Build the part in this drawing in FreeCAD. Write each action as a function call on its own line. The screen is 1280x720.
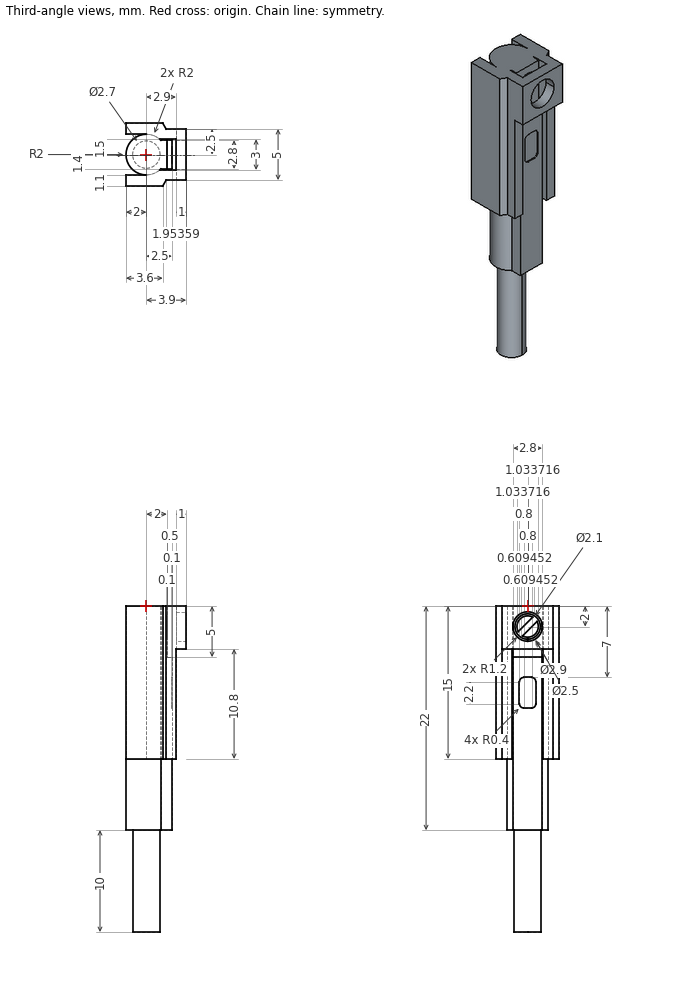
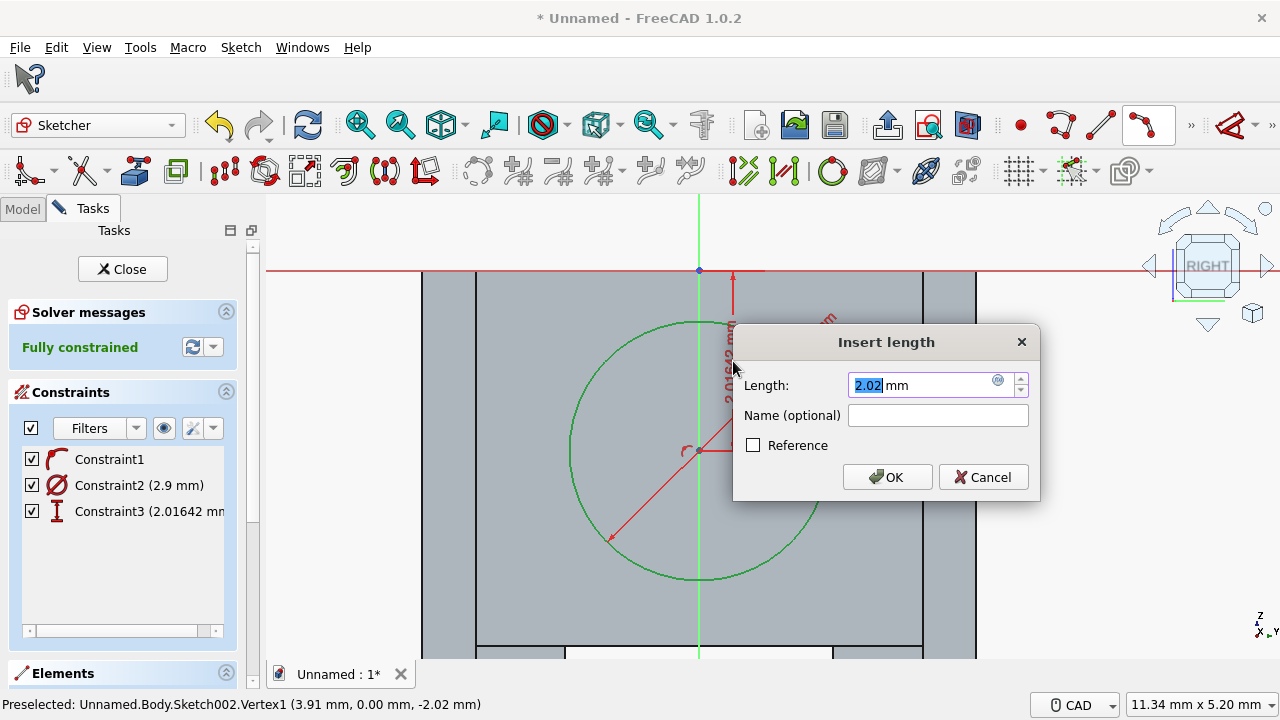
text(2)
key(Return)
key(Escape)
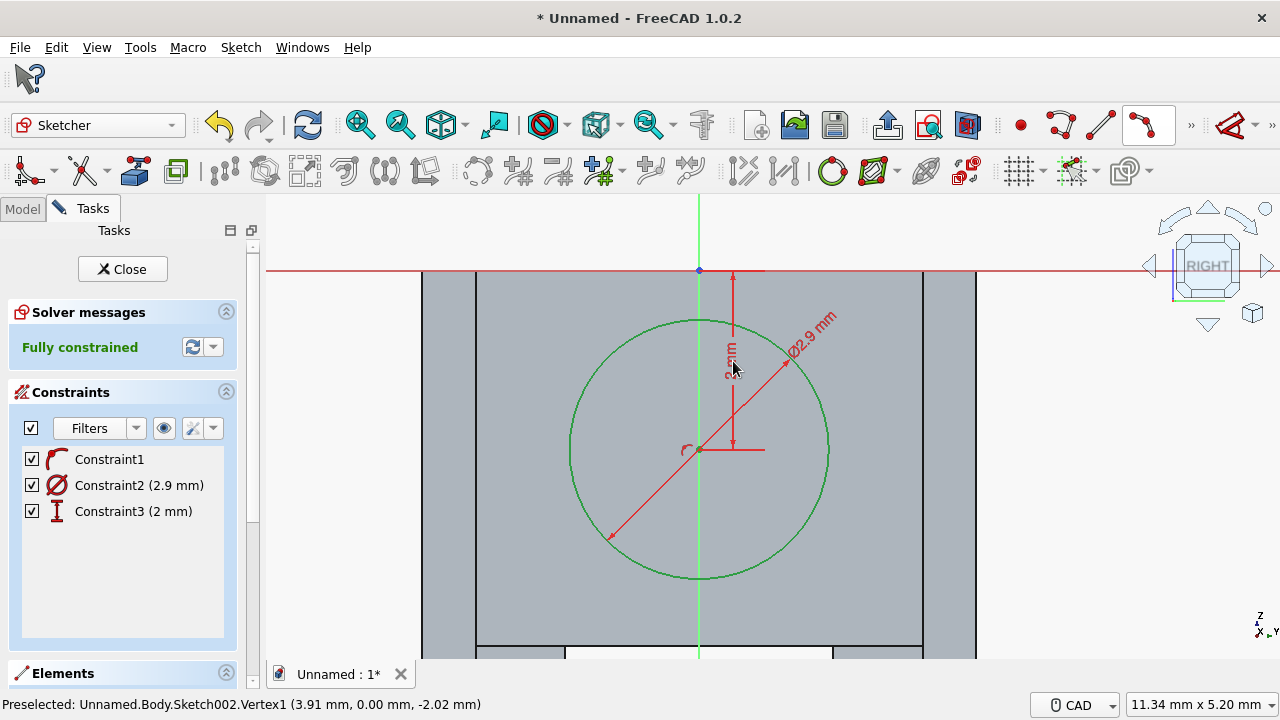
click(123, 269)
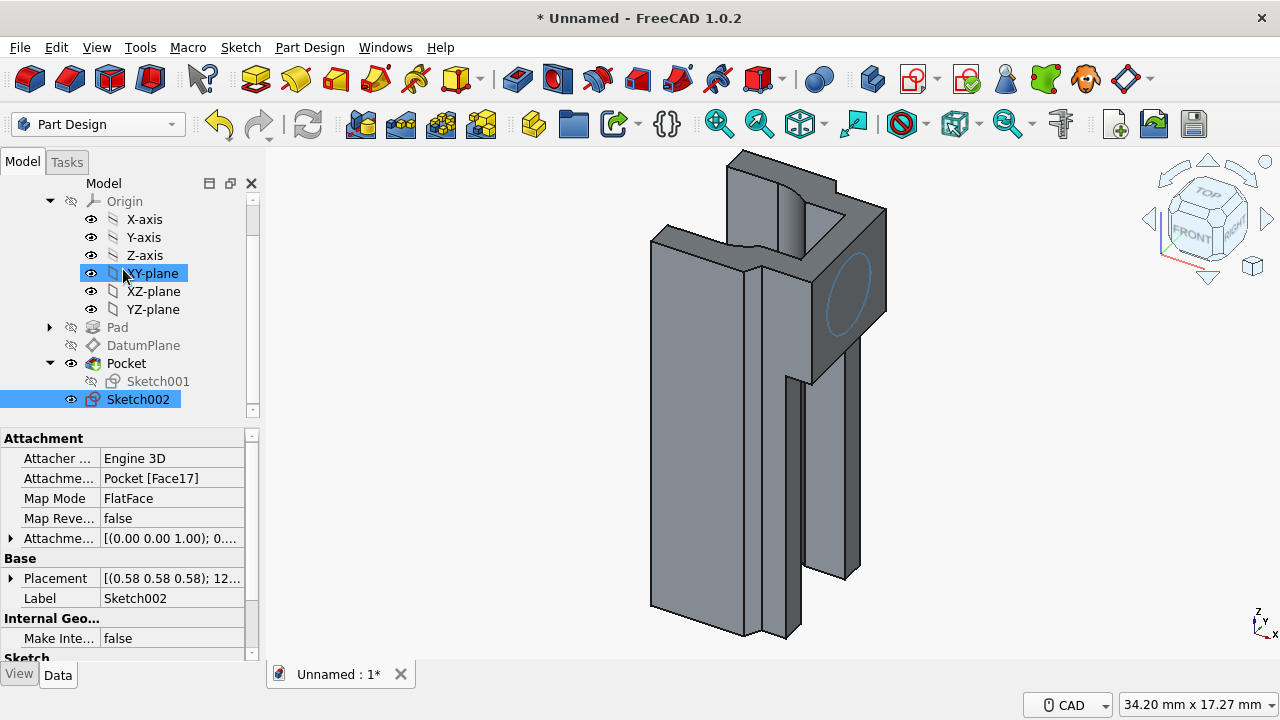
click(518, 80)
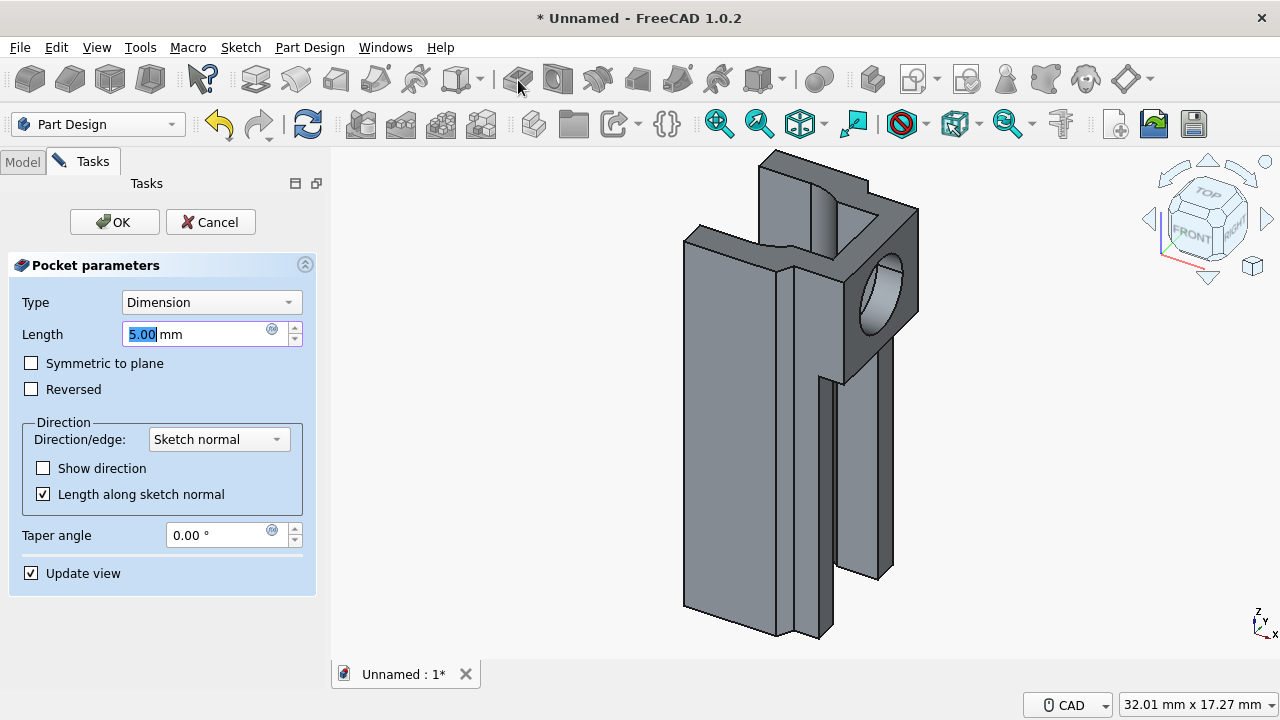
text(1)
key(Tab)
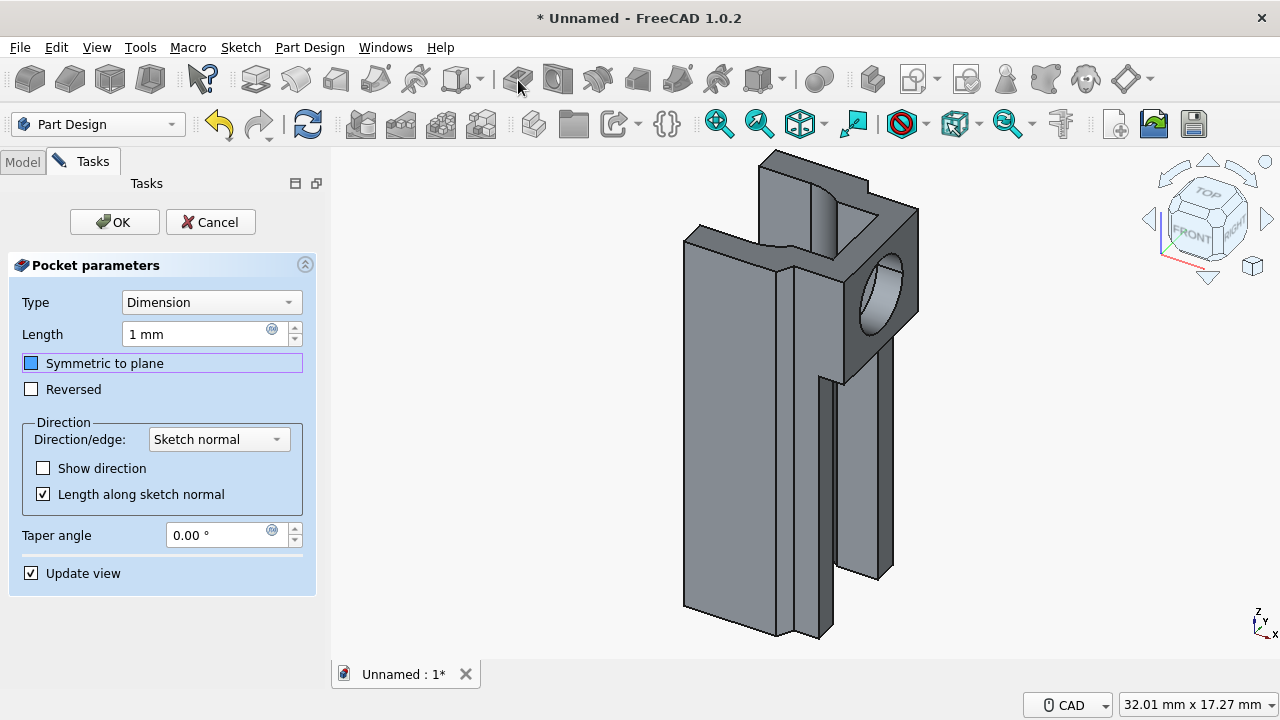
click(115, 222)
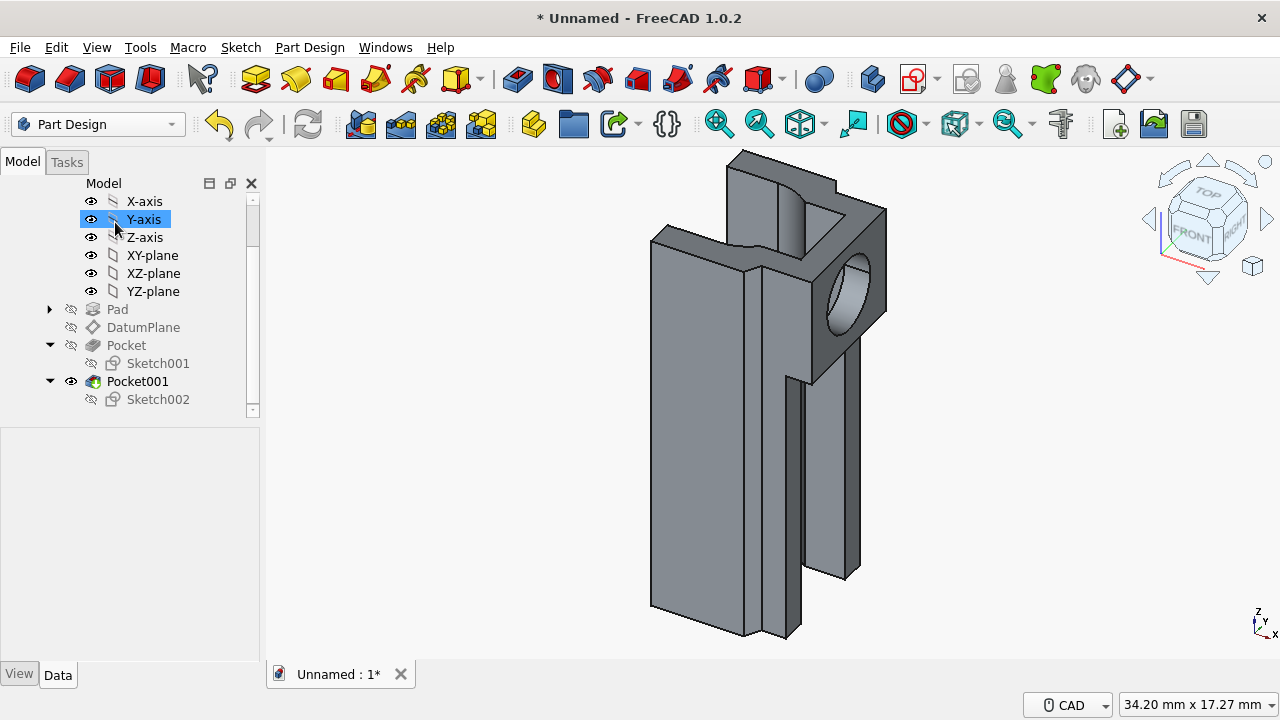
click(812, 181)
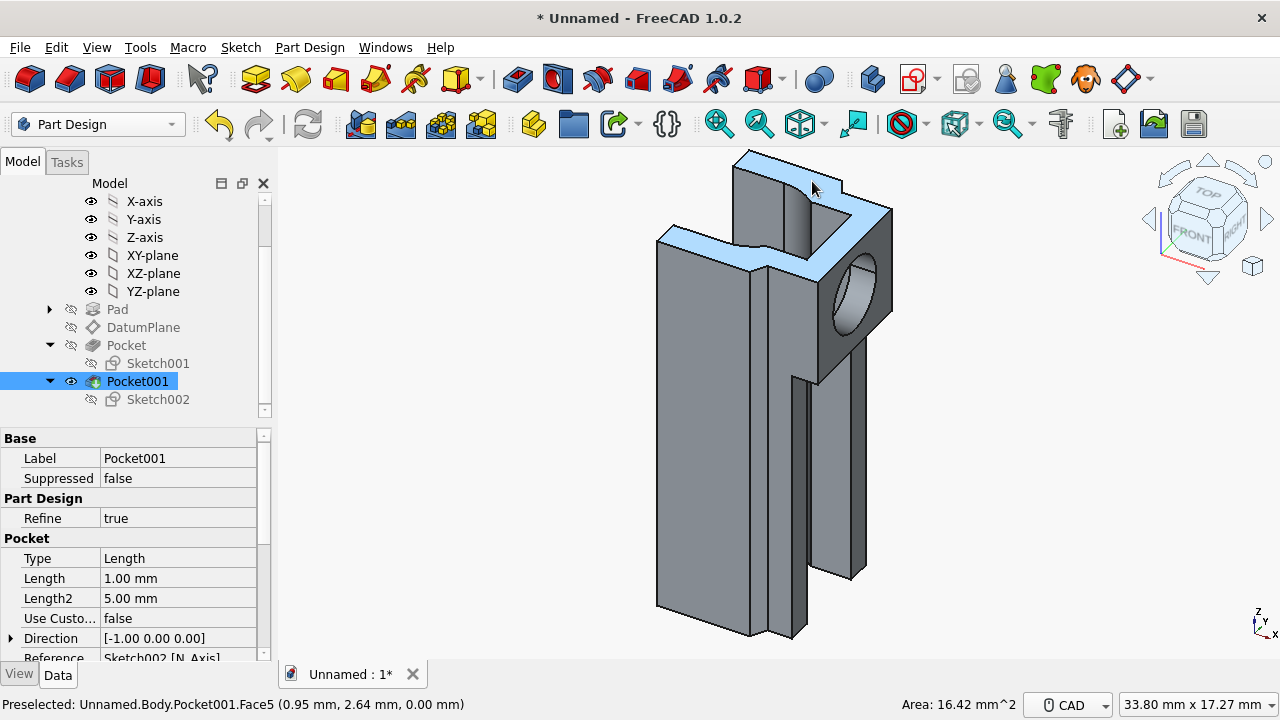
click(914, 80)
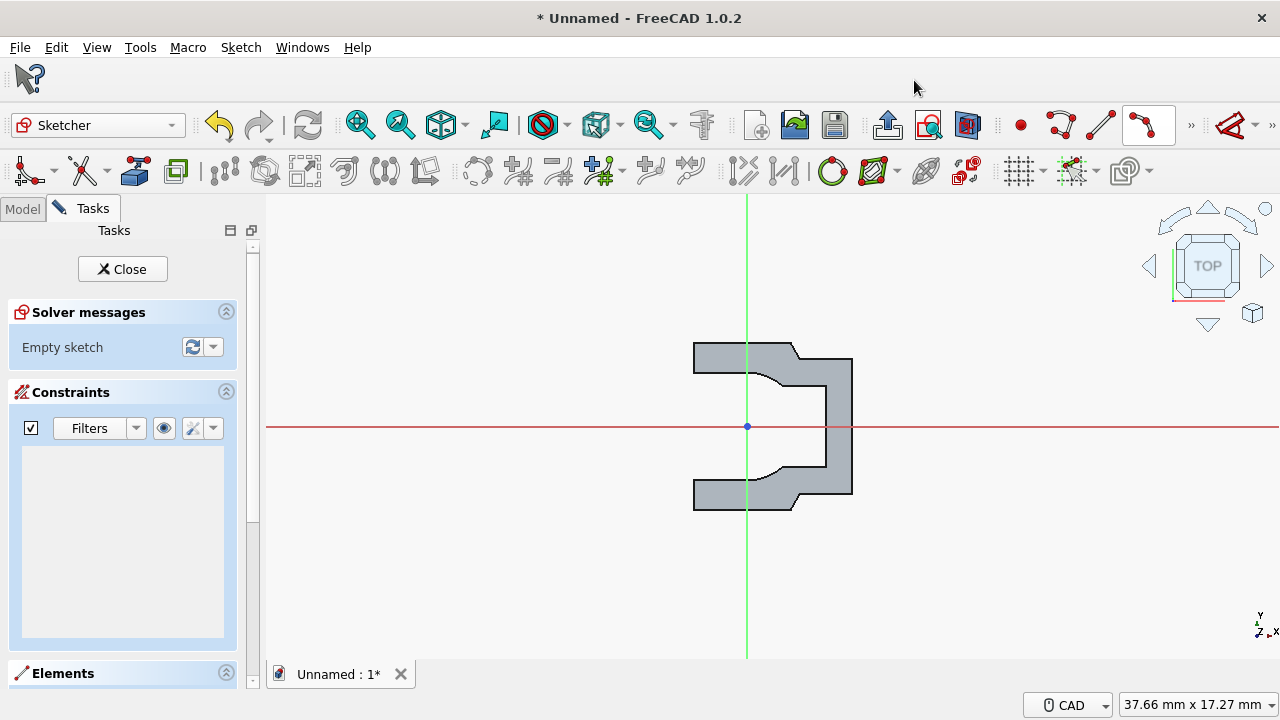
scroll(770, 426, up, 7)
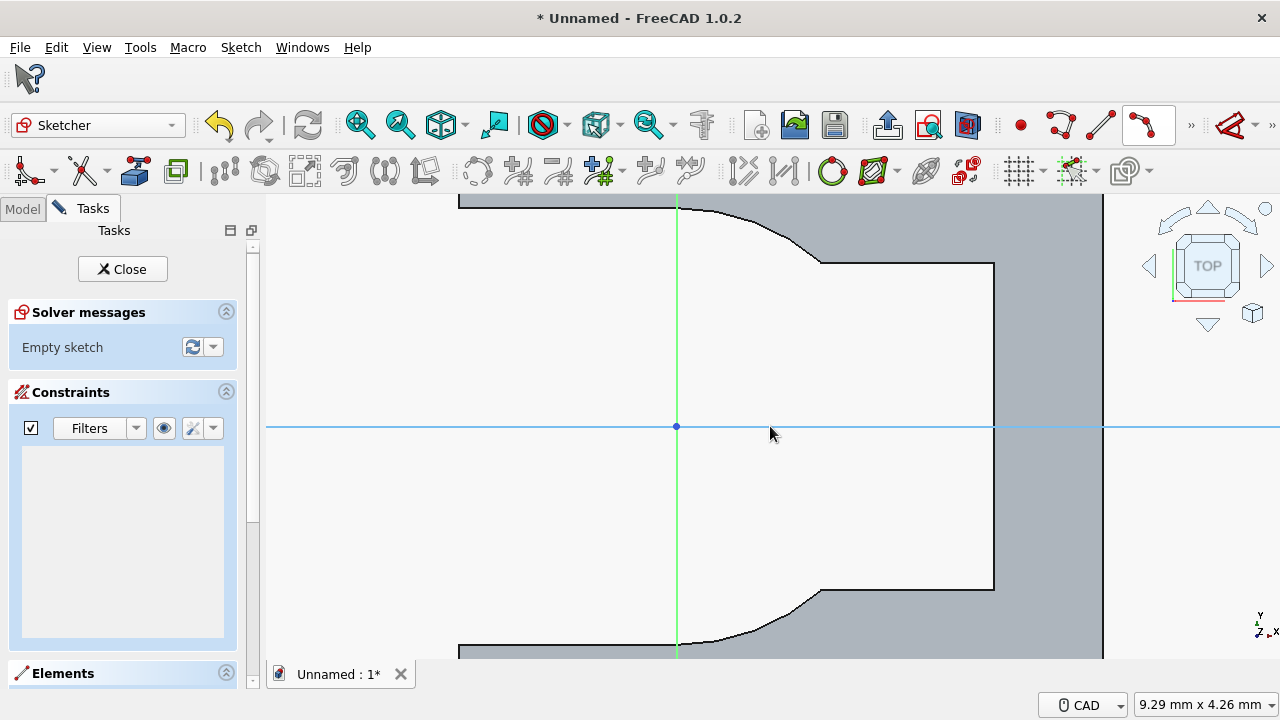
click(1062, 126)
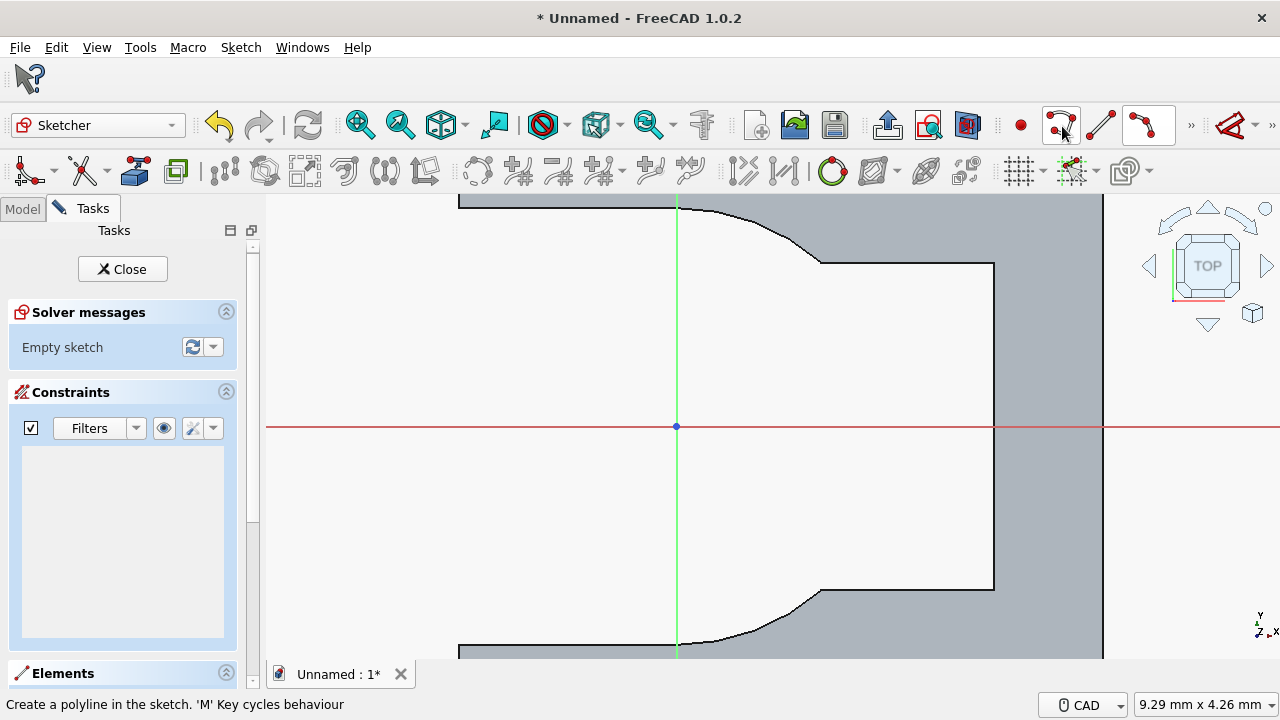
click(833, 579)
click(950, 579)
click(950, 274)
click(833, 274)
right_click(833, 274)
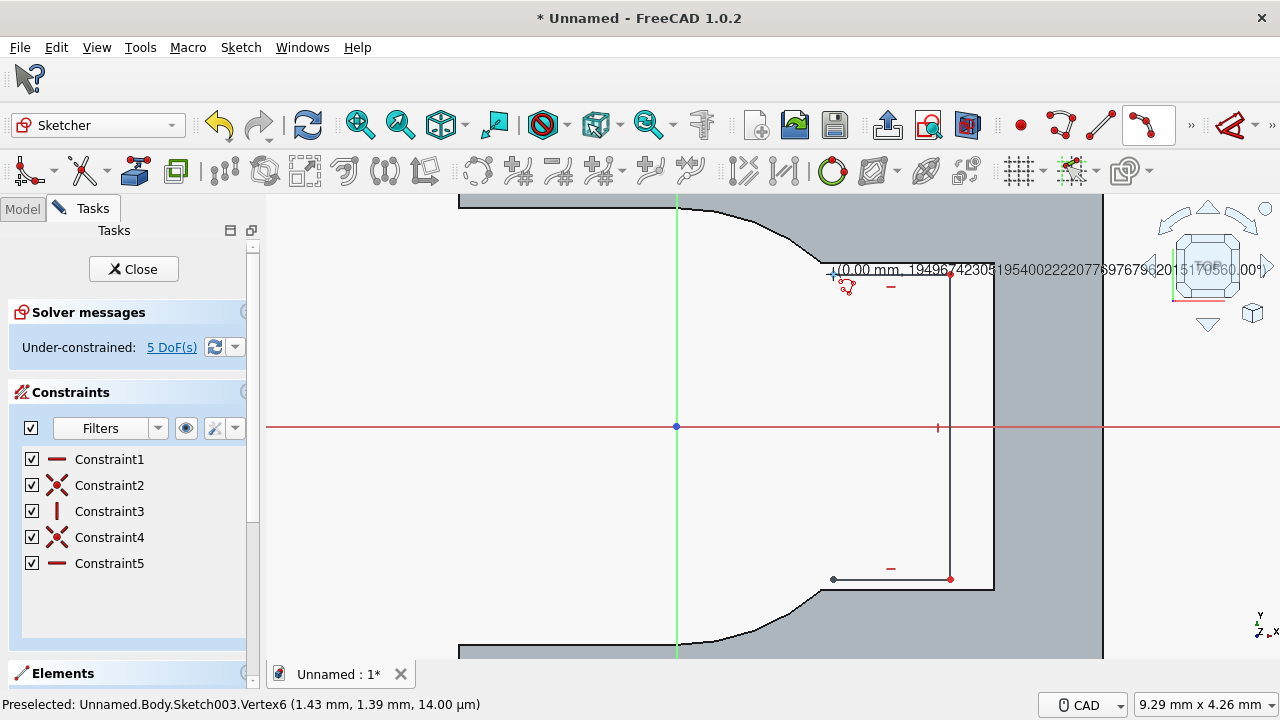
click(1142, 126)